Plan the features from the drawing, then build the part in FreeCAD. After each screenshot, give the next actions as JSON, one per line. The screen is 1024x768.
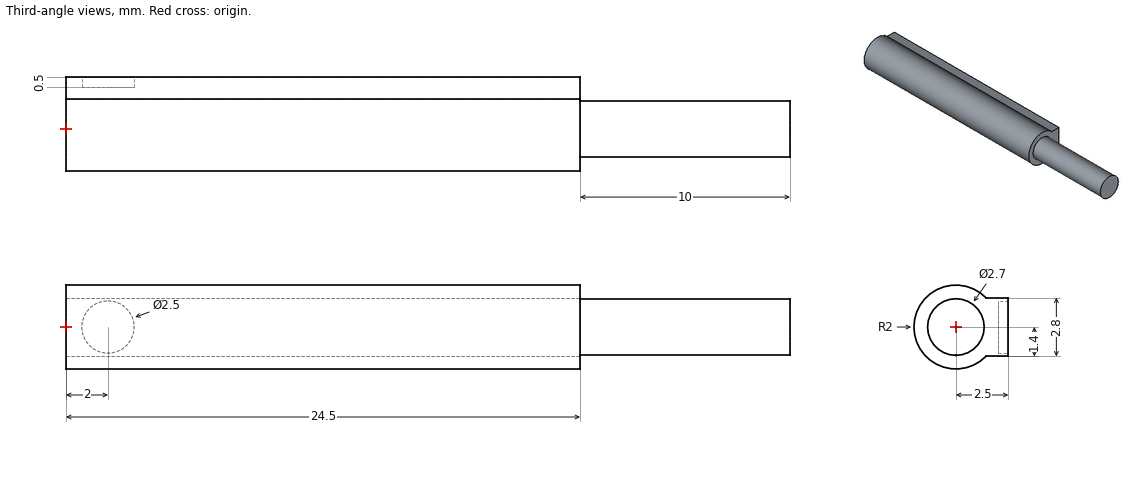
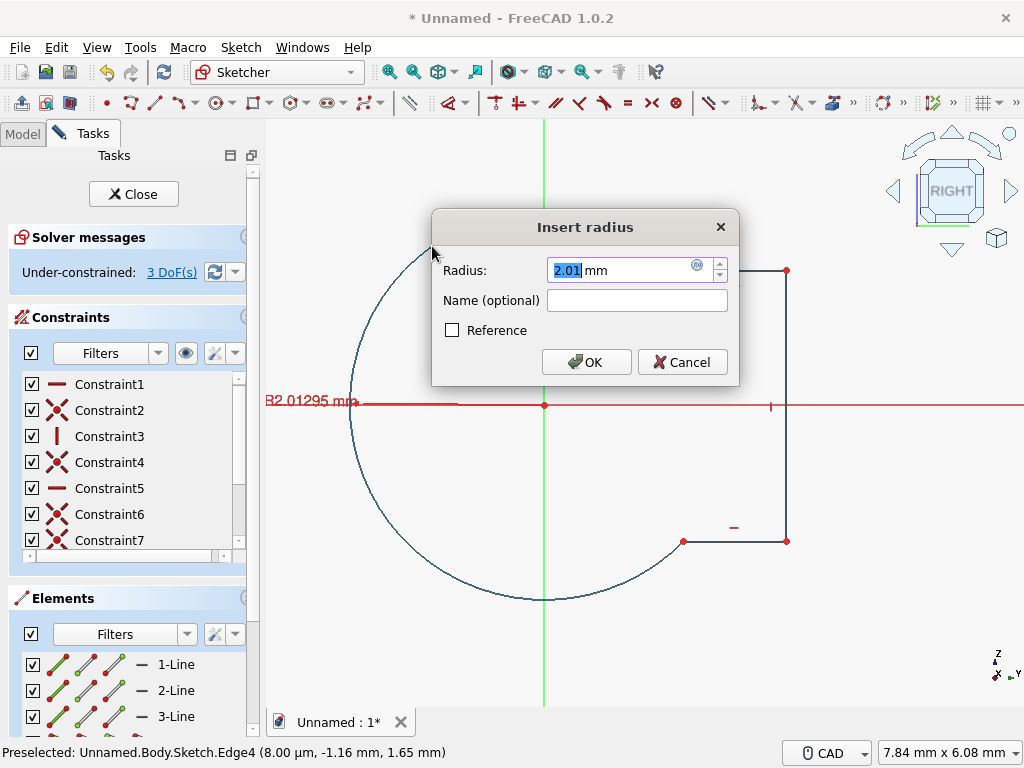
{"action": "type", "text": "2"}
{"action": "key", "text": "Return"}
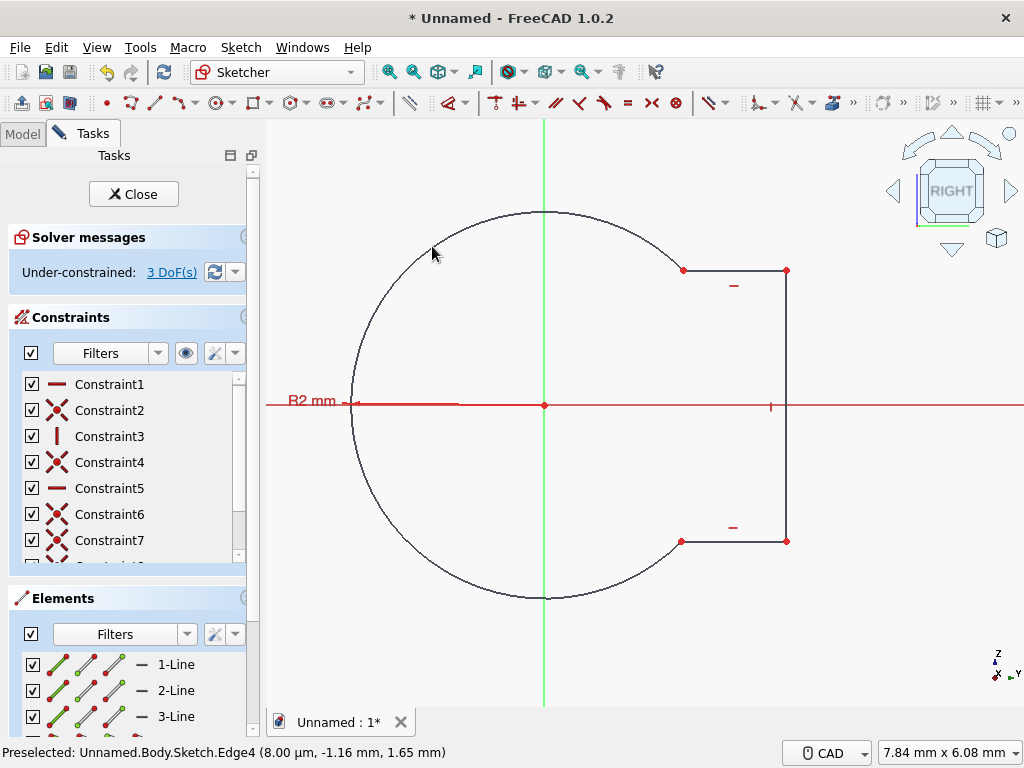
{"action": "left_click", "coordinate": [786, 461]}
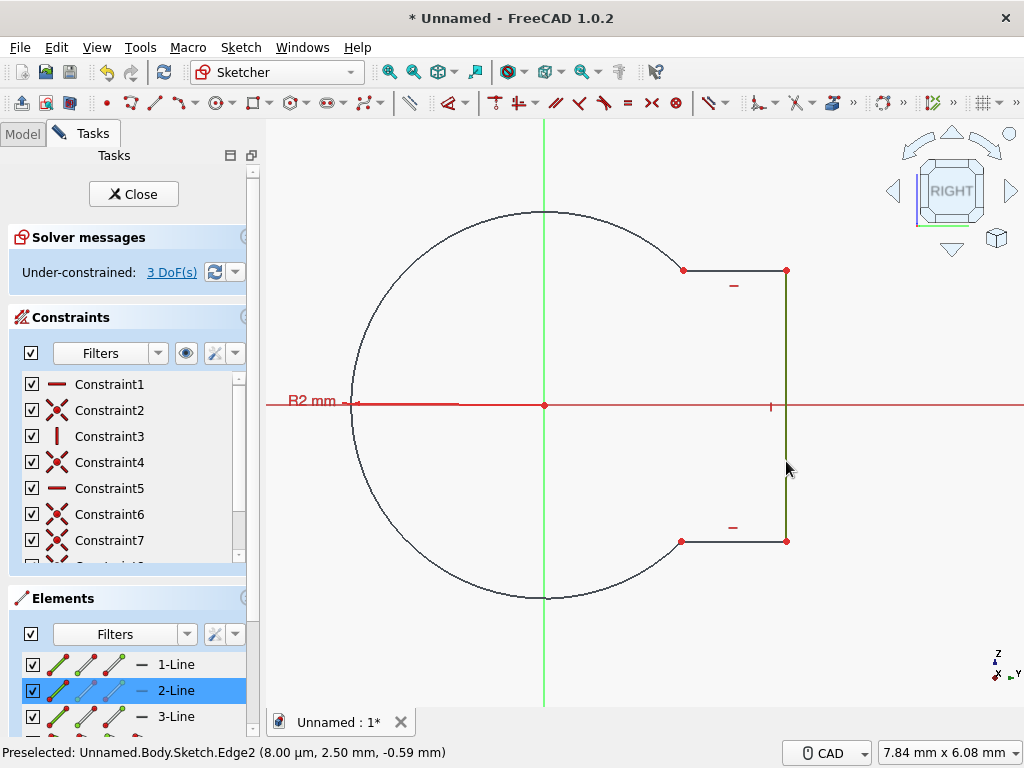
{"action": "key", "text": "i"}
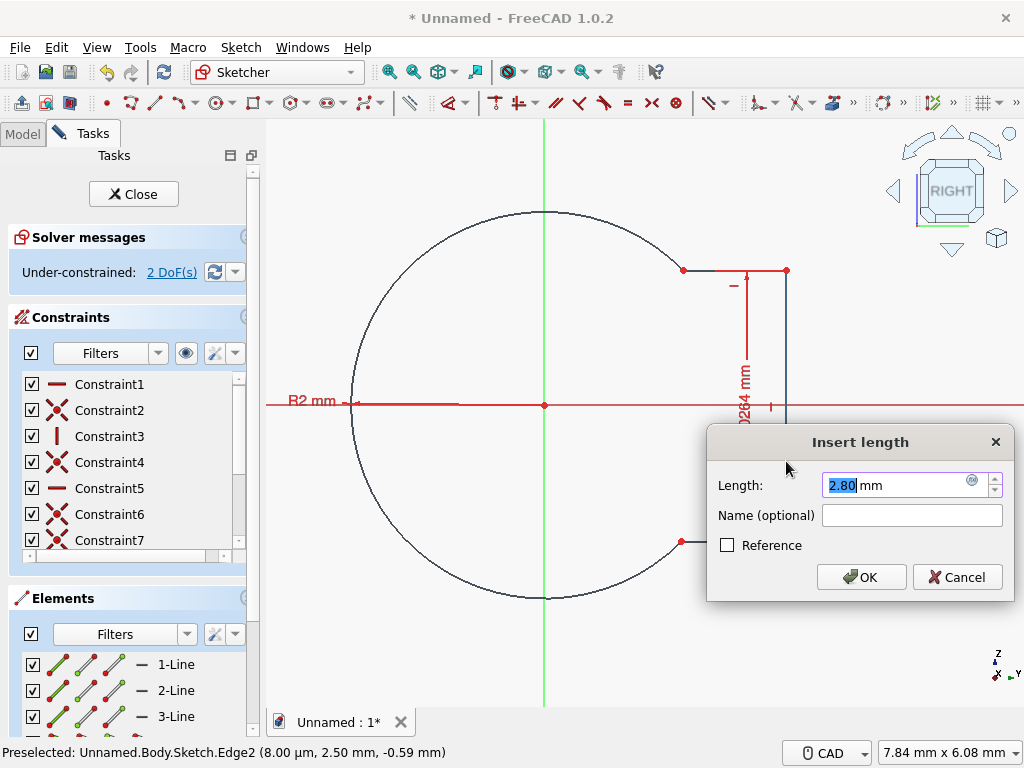
{"action": "type", "text": "2.8"}
{"action": "key", "text": "Return"}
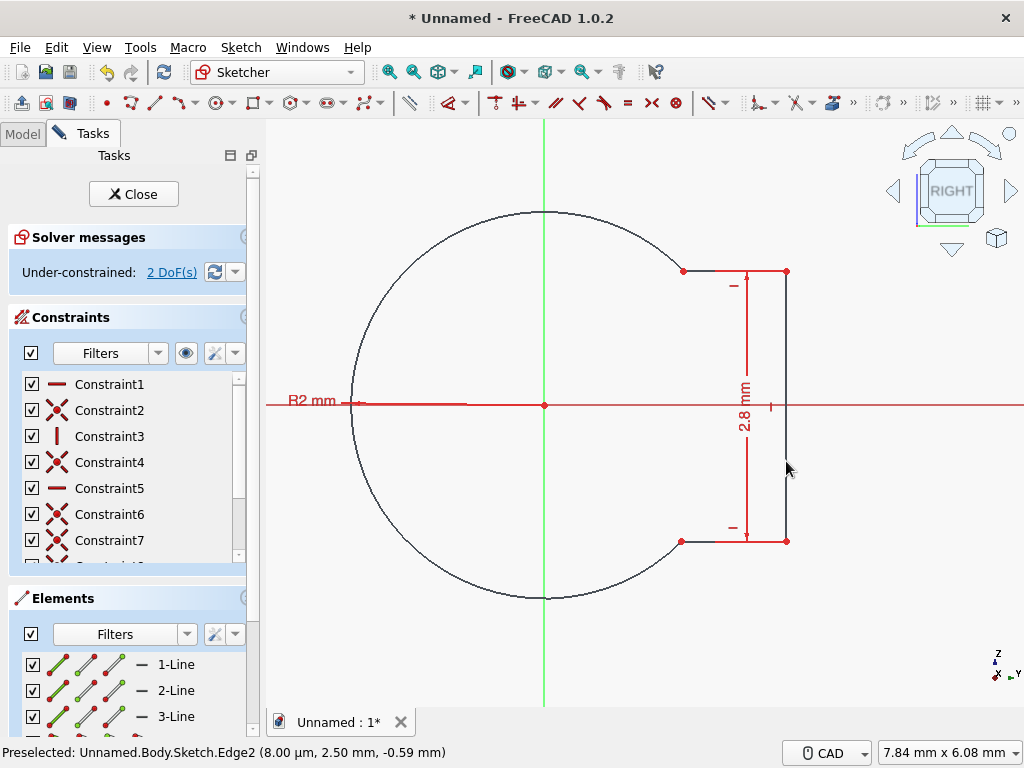
{"action": "left_click", "coordinate": [681, 542]}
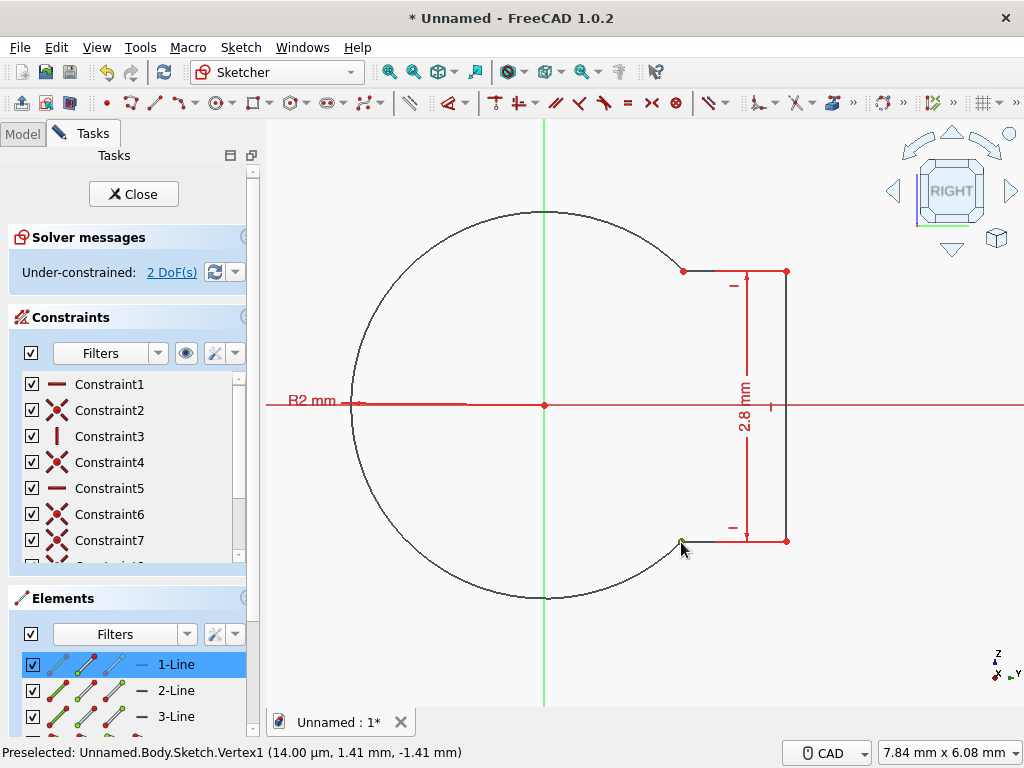
{"action": "key", "text": "i"}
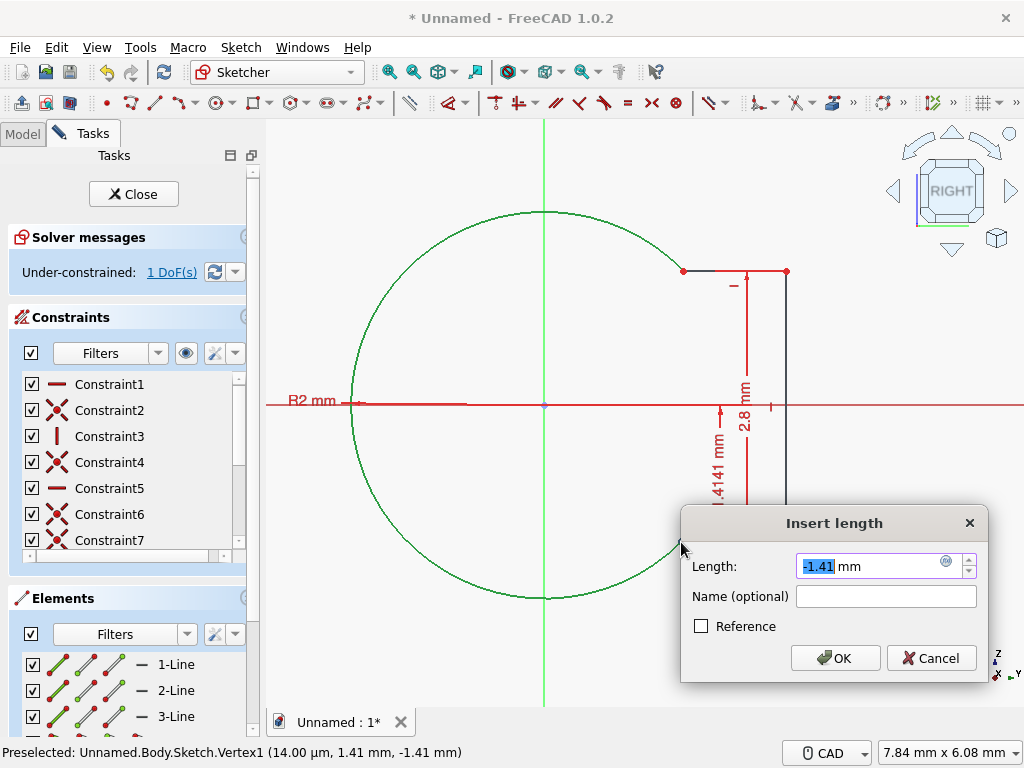
{"action": "type", "text": "-1.4"}
{"action": "key", "text": "Return"}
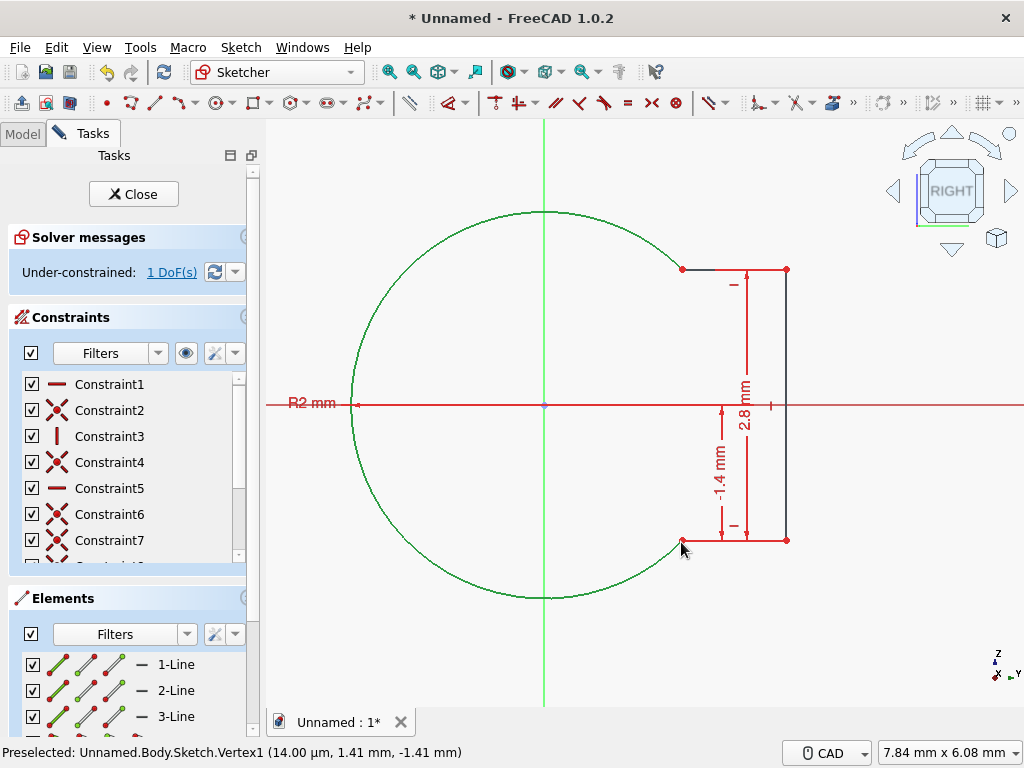
{"action": "left_click", "coordinate": [786, 541]}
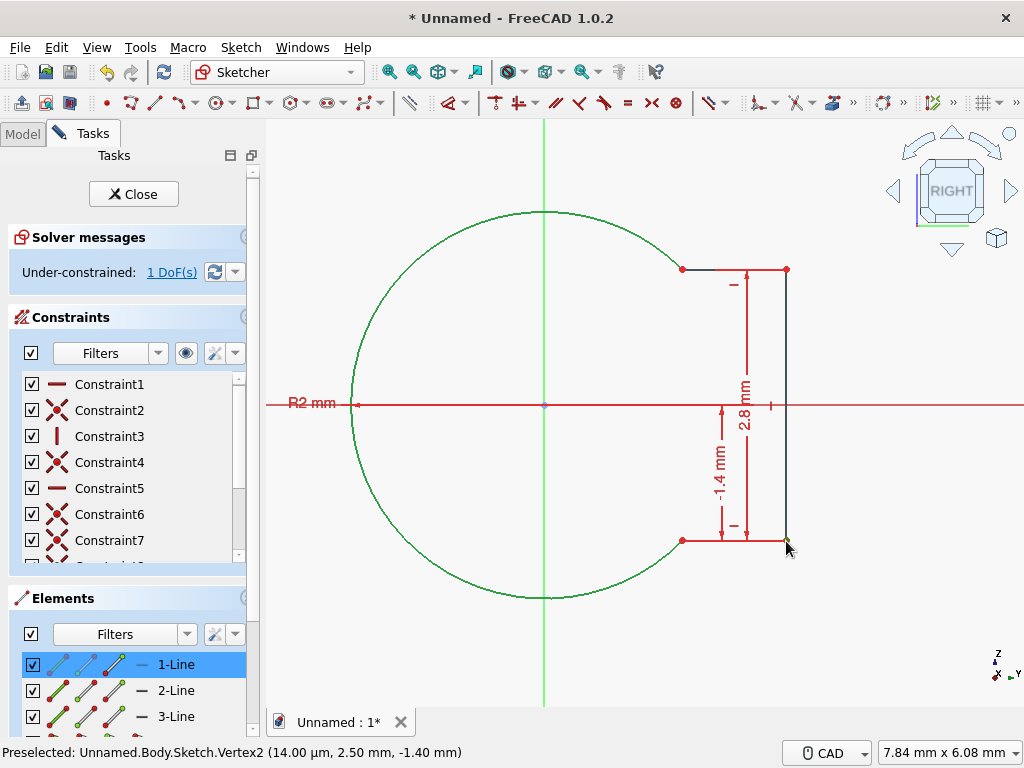
{"action": "left_click", "coordinate": [468, 104]}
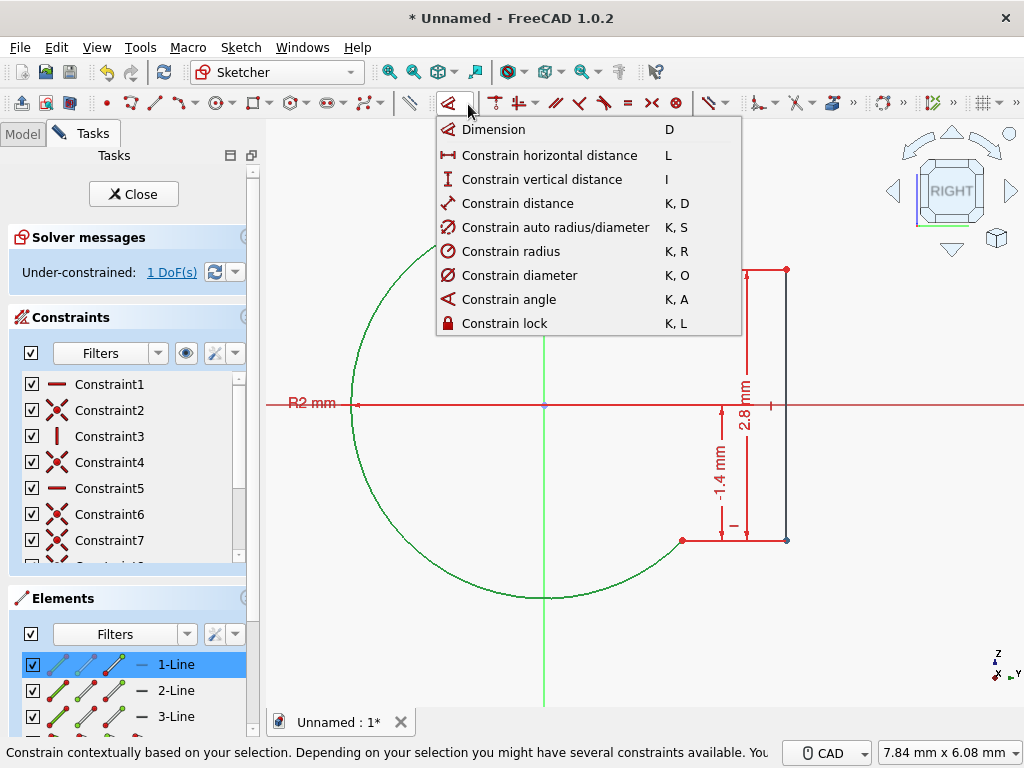
{"action": "left_click", "coordinate": [589, 155]}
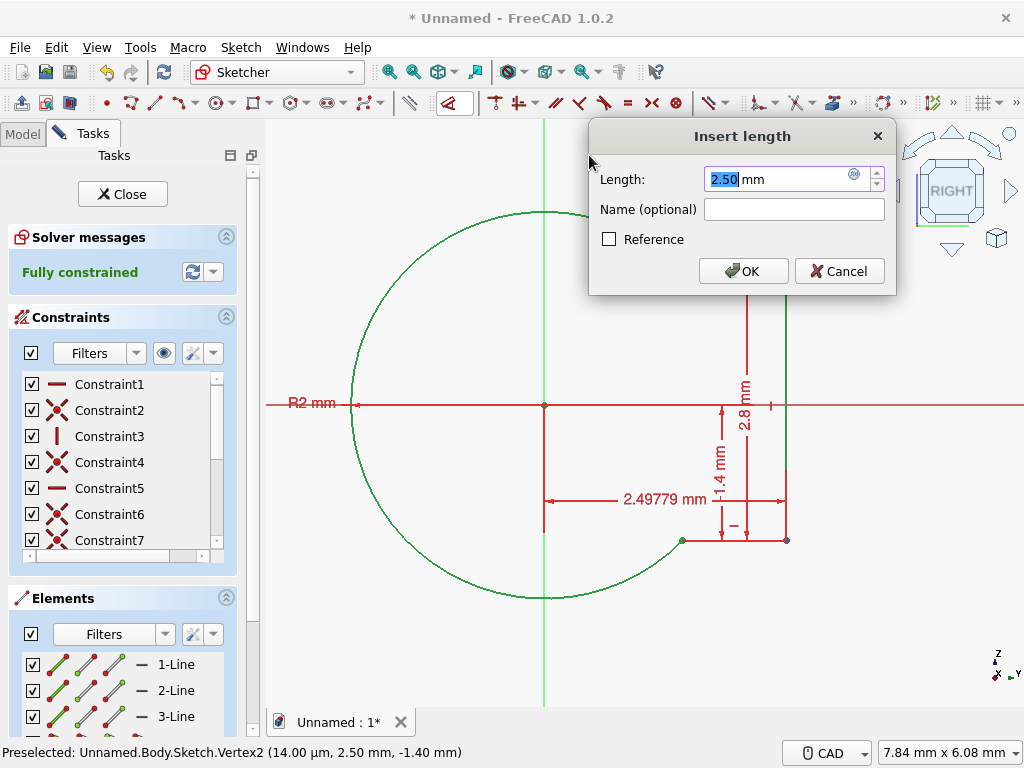
{"action": "type", "text": "2.5"}
{"action": "key", "text": "Return"}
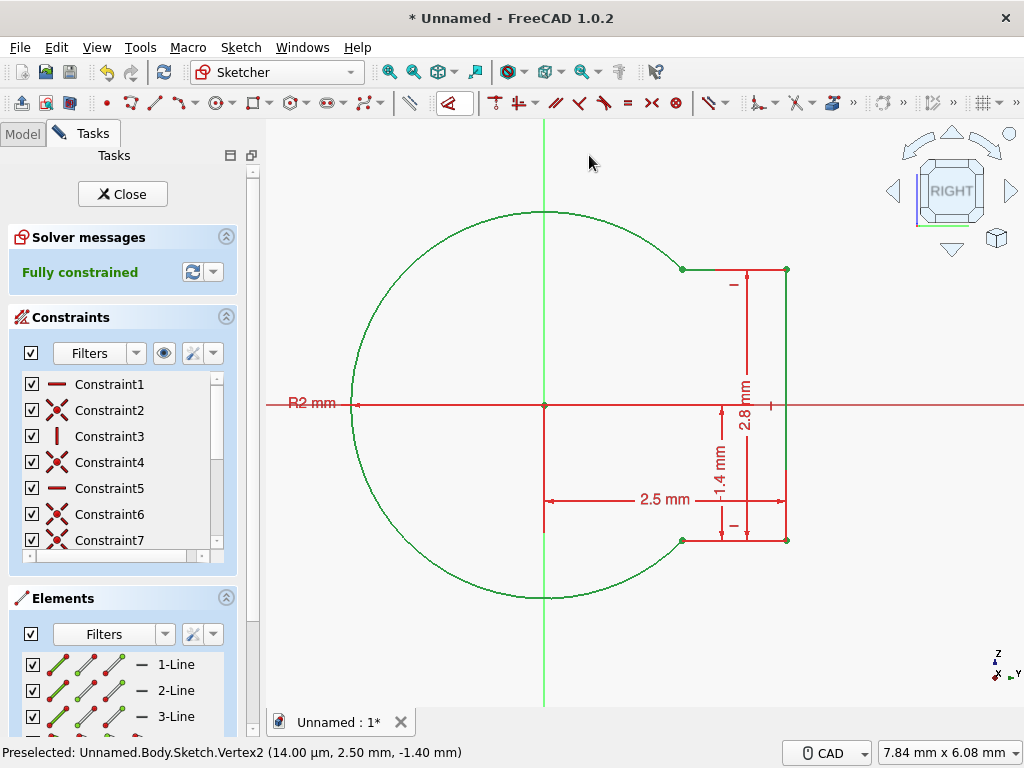
{"action": "left_click", "coordinate": [123, 194]}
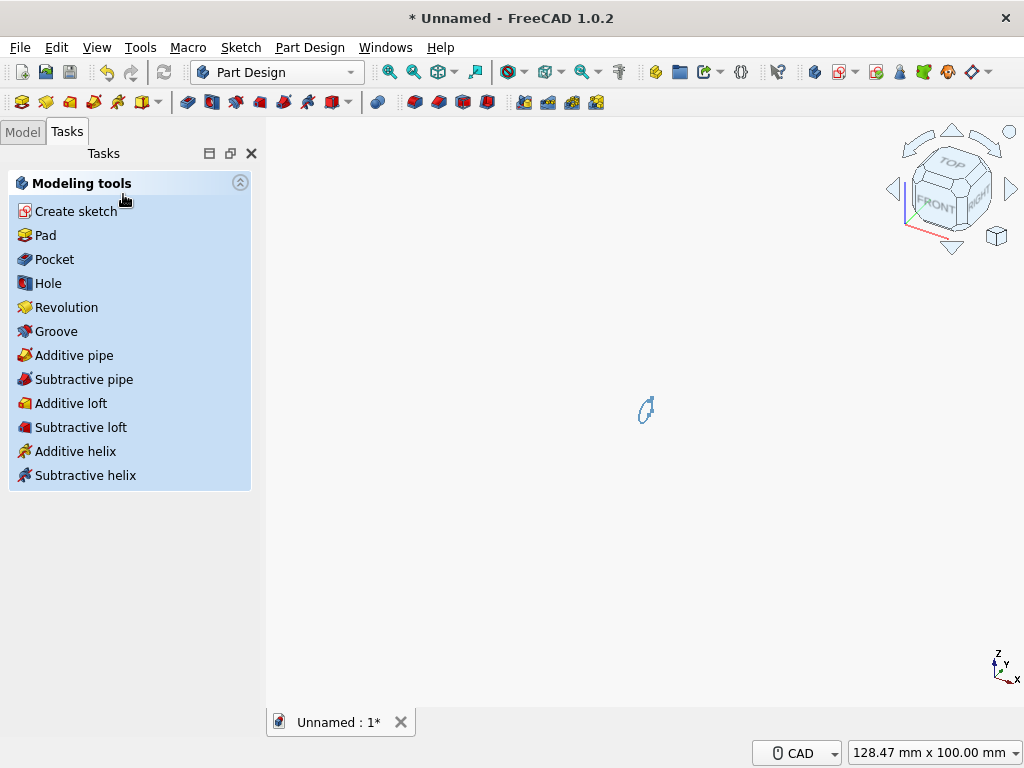
{"action": "left_click", "coordinate": [22, 102]}